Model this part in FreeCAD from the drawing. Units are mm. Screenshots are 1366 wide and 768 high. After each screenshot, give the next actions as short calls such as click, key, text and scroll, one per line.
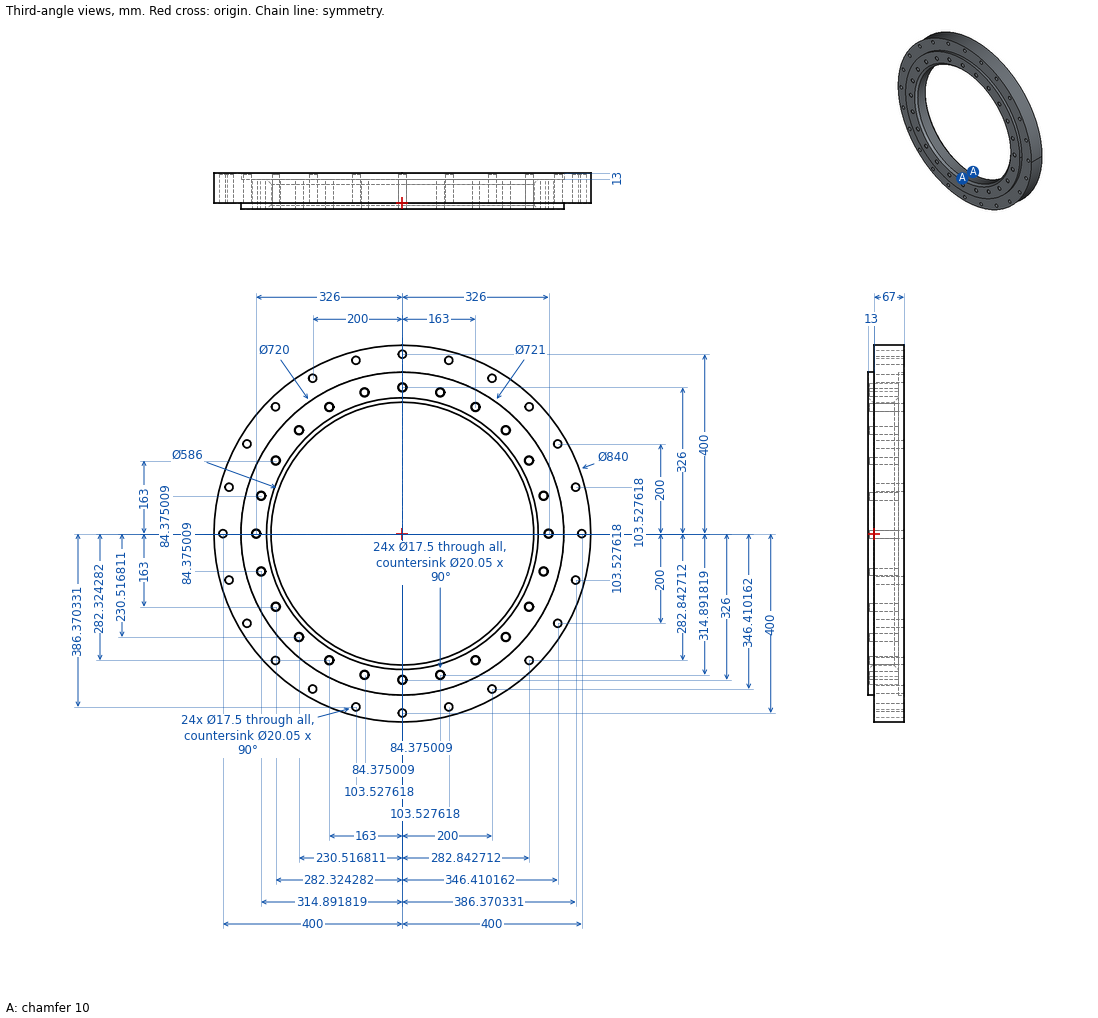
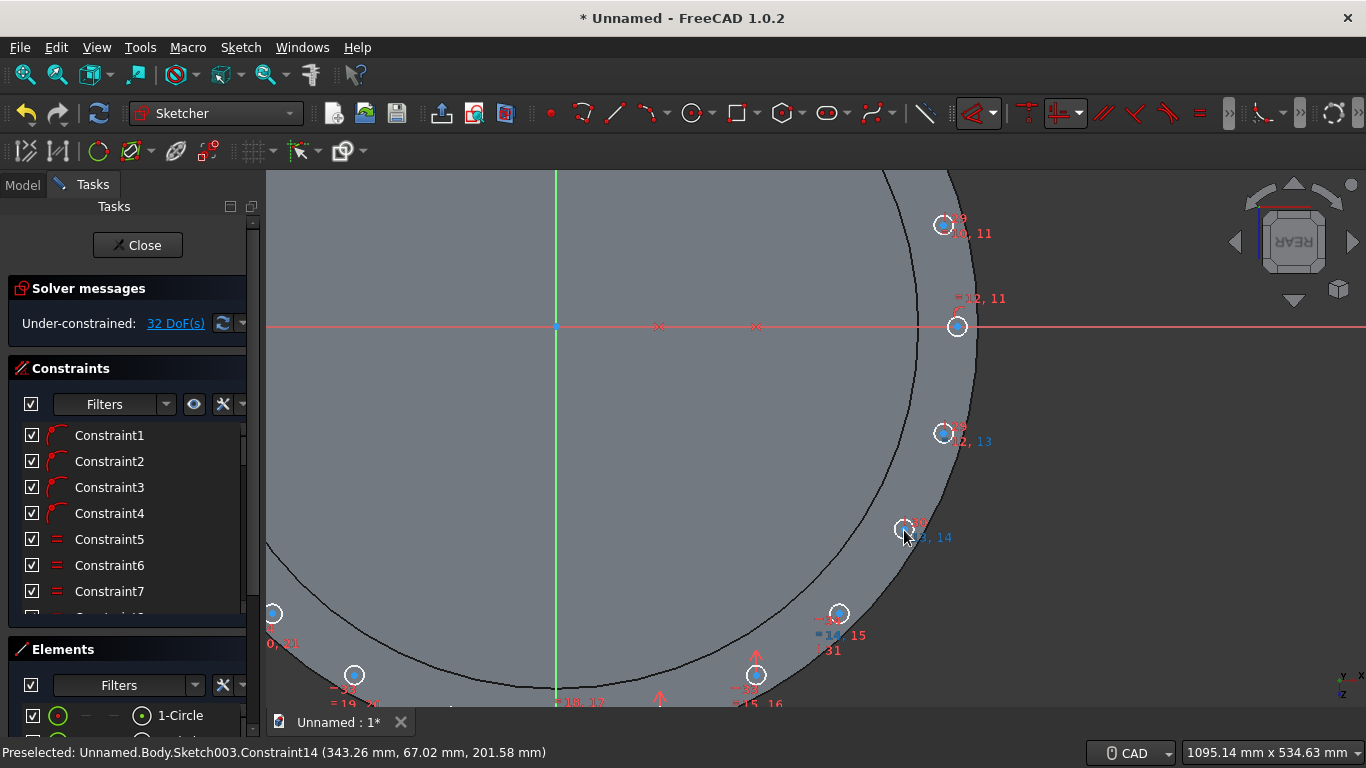
scroll(904, 529, up, 4)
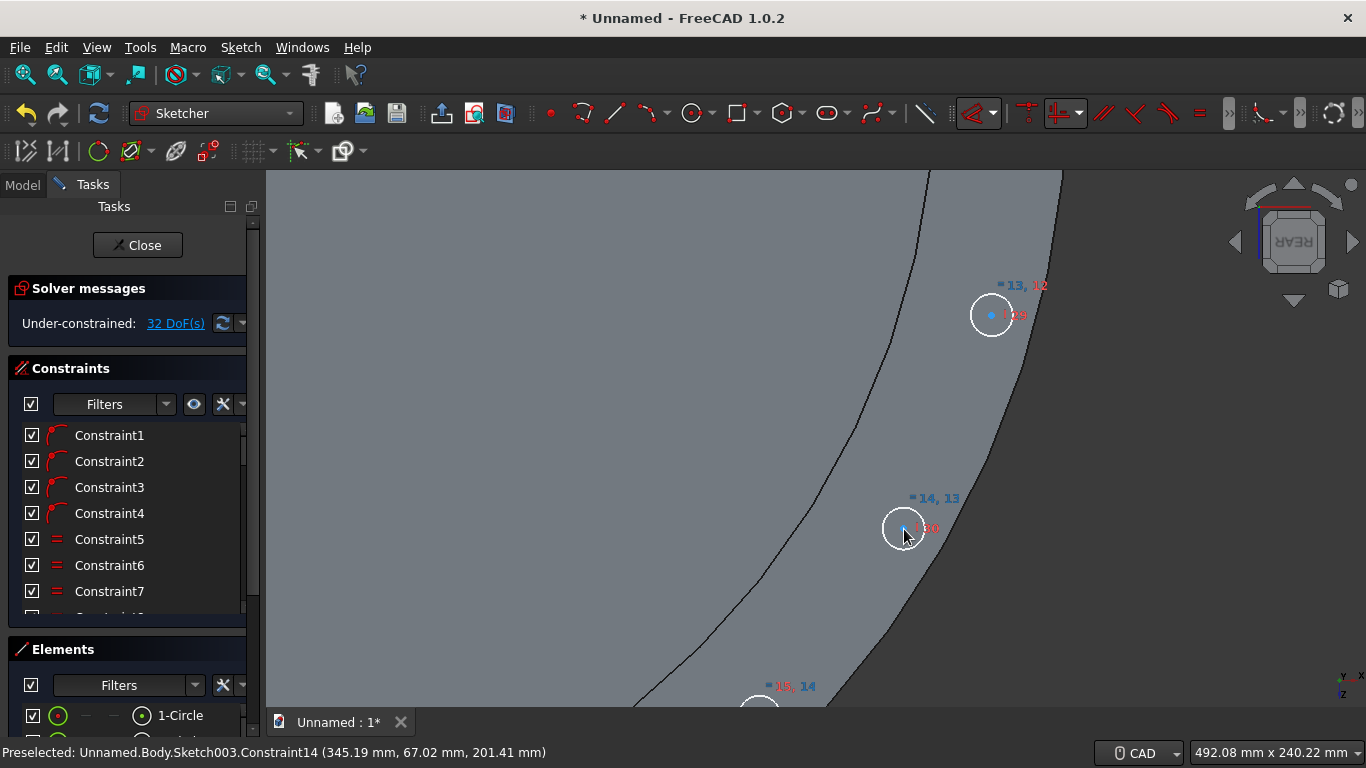
click(904, 529)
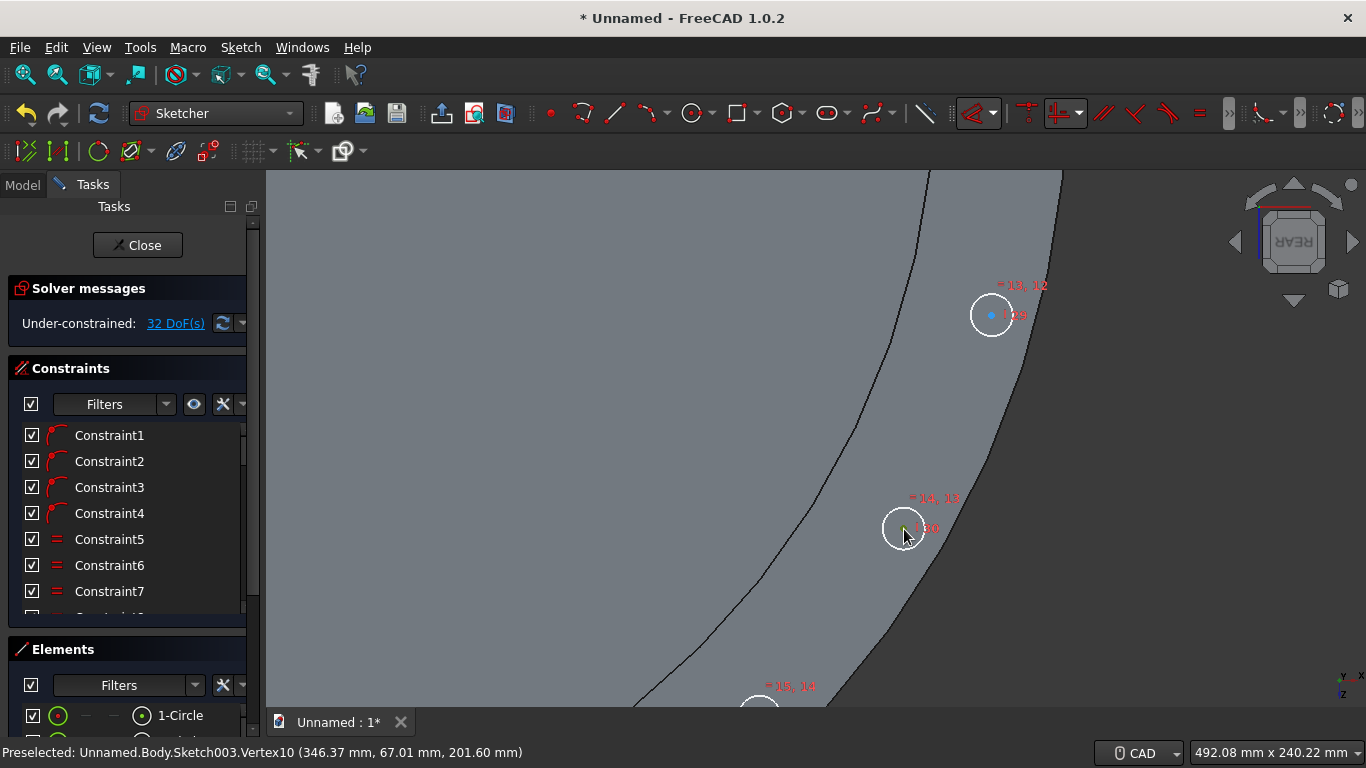
scroll(904, 530, down, 8)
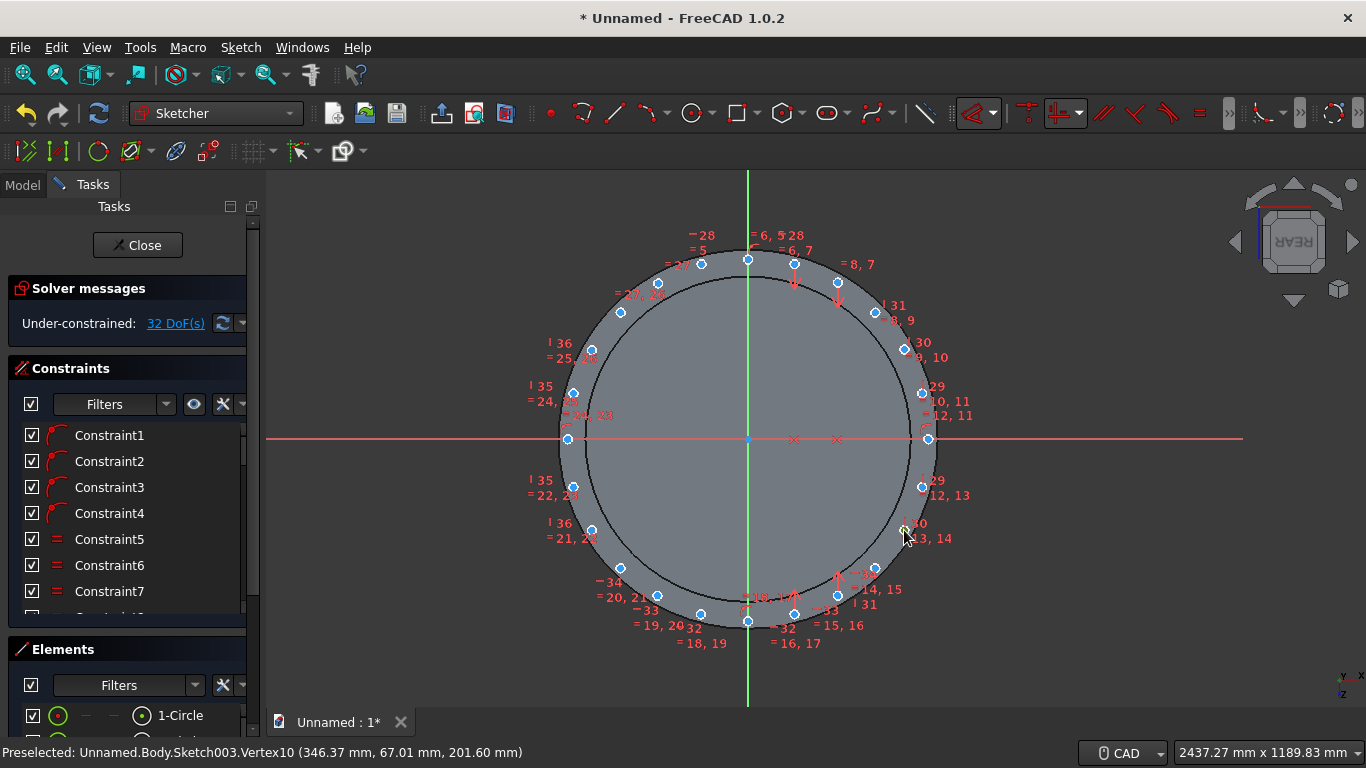
click(592, 530)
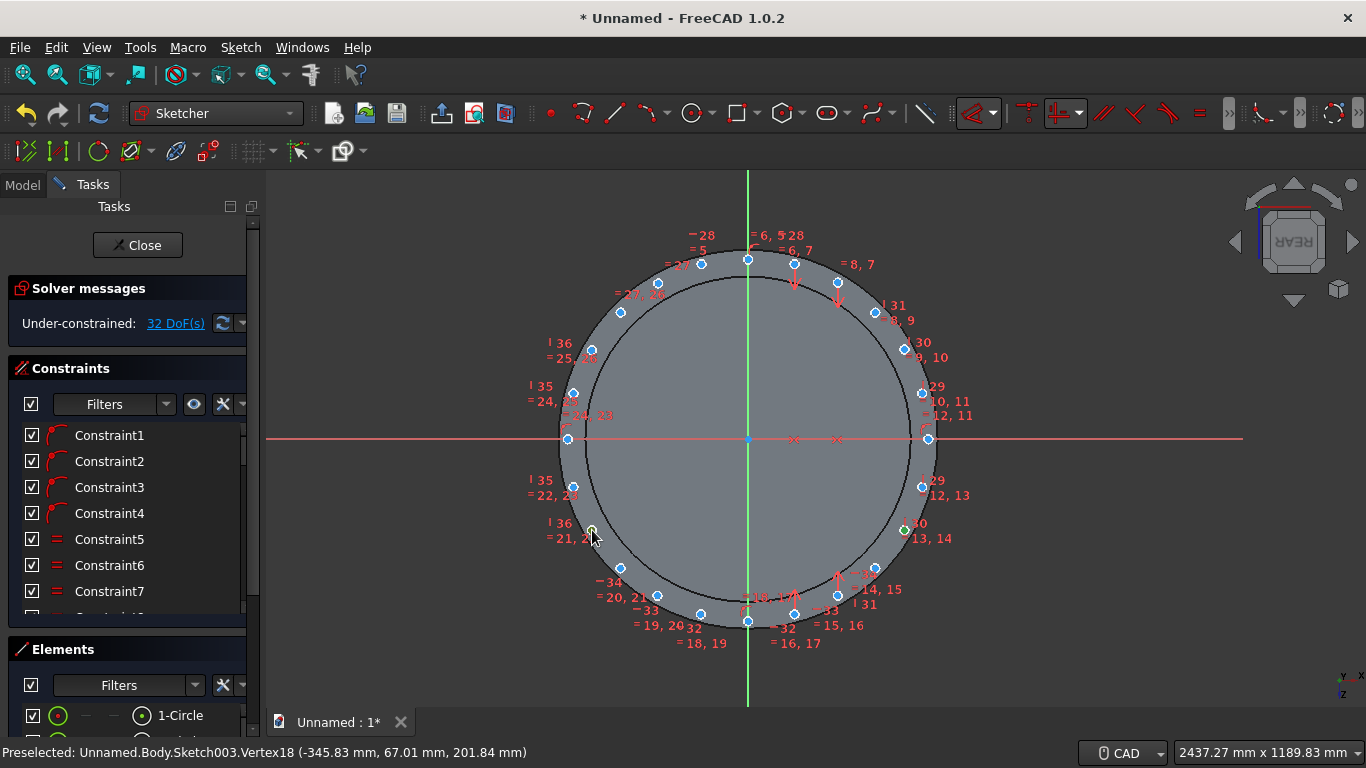
click(748, 576)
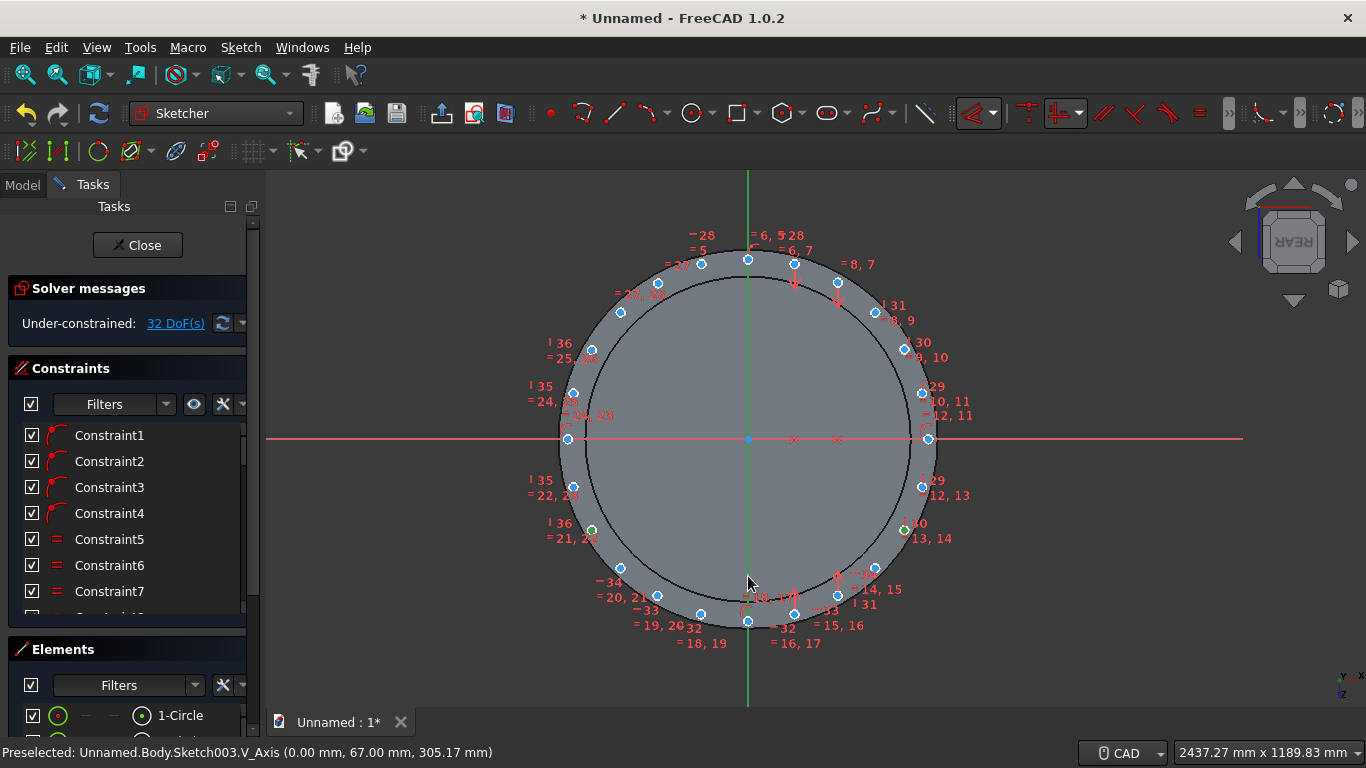
key(s)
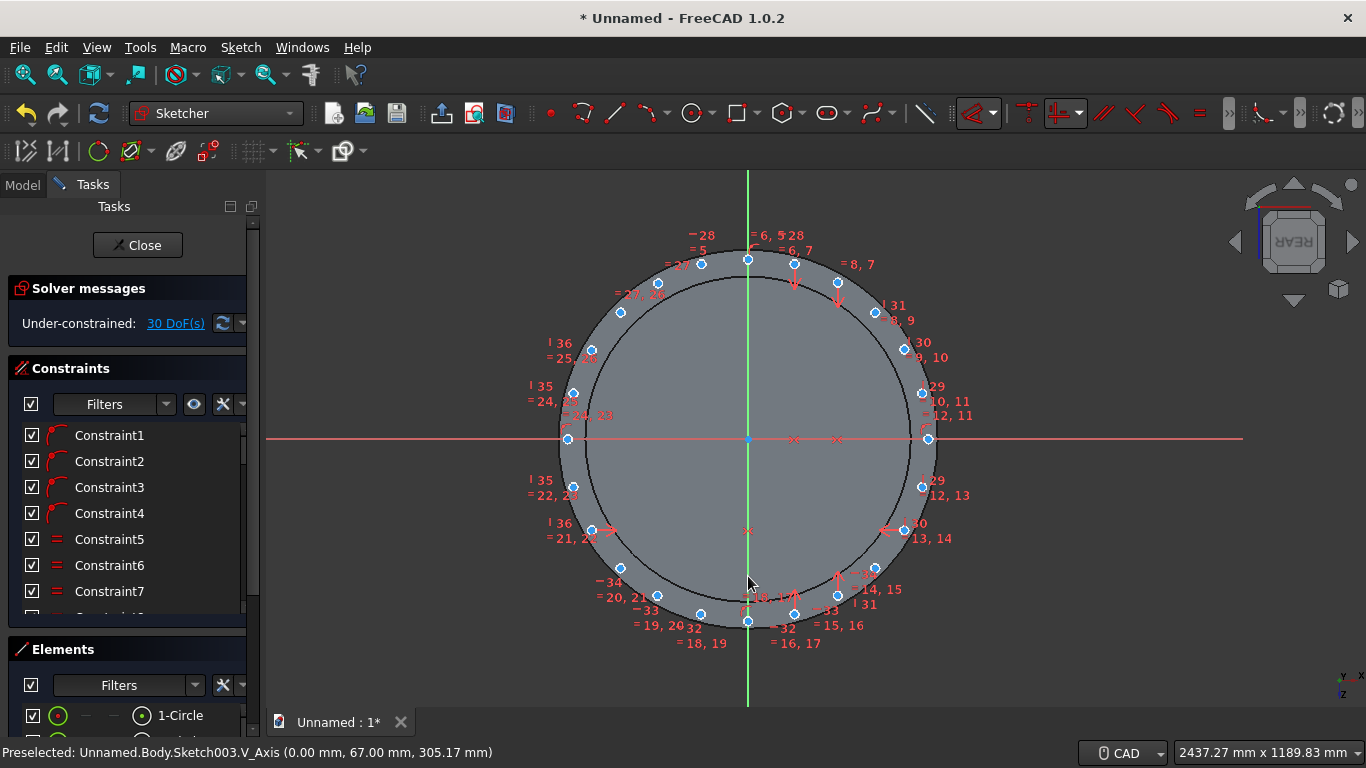
scroll(922, 487, up, 4)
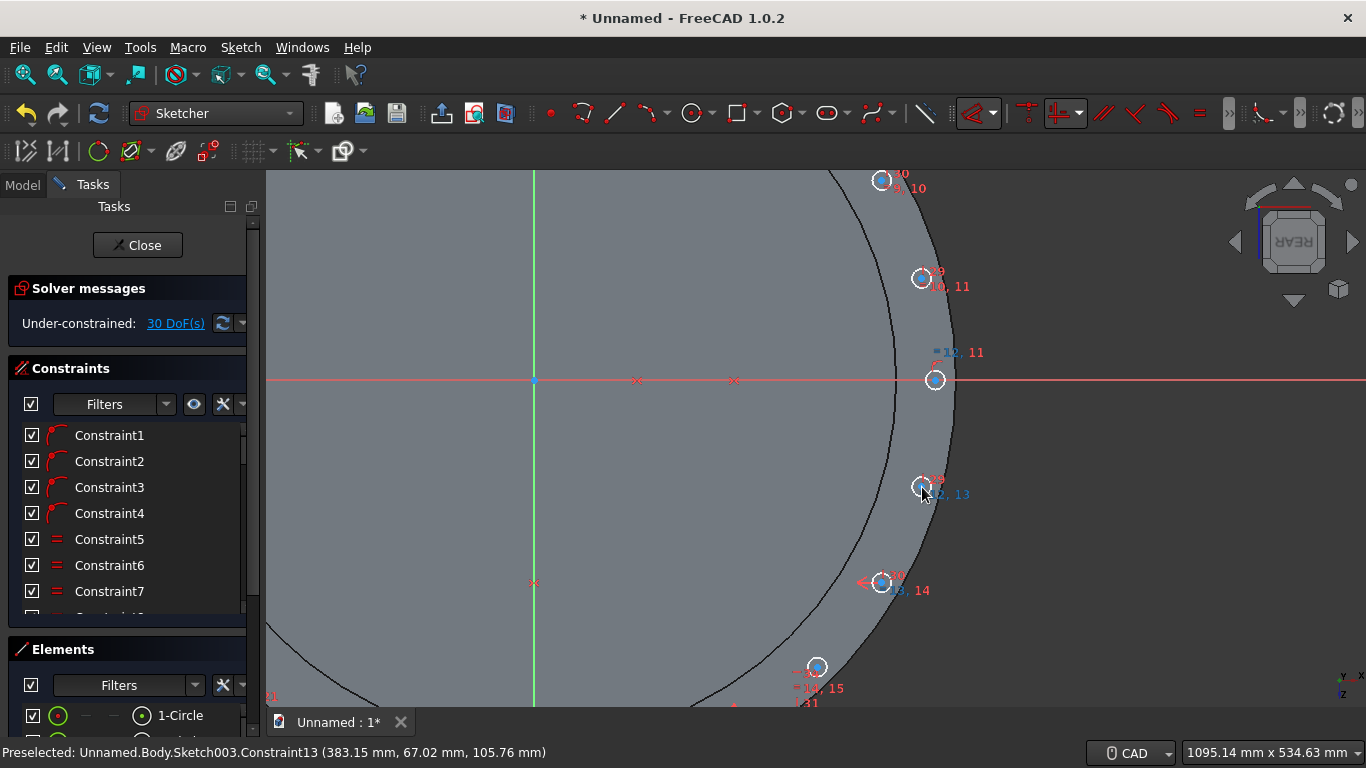
scroll(922, 487, up, 4)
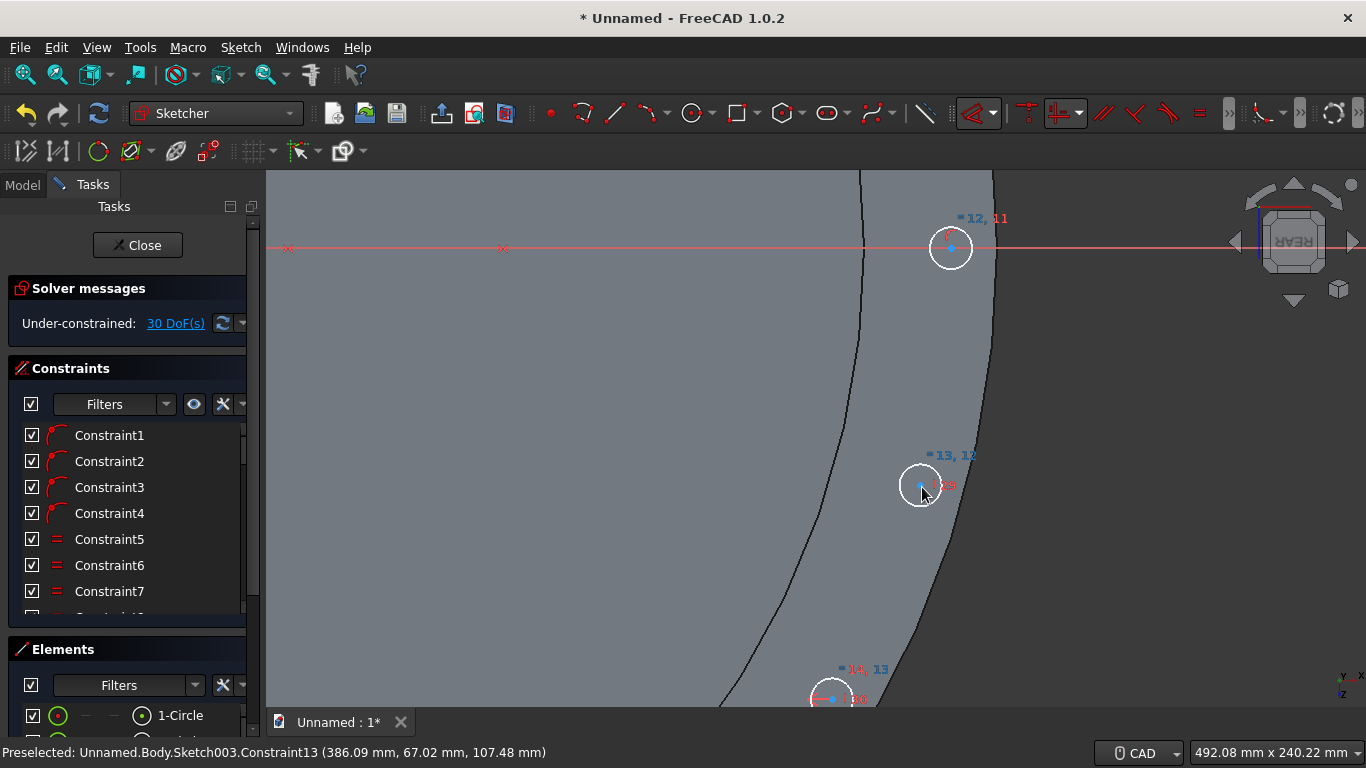
click(921, 485)